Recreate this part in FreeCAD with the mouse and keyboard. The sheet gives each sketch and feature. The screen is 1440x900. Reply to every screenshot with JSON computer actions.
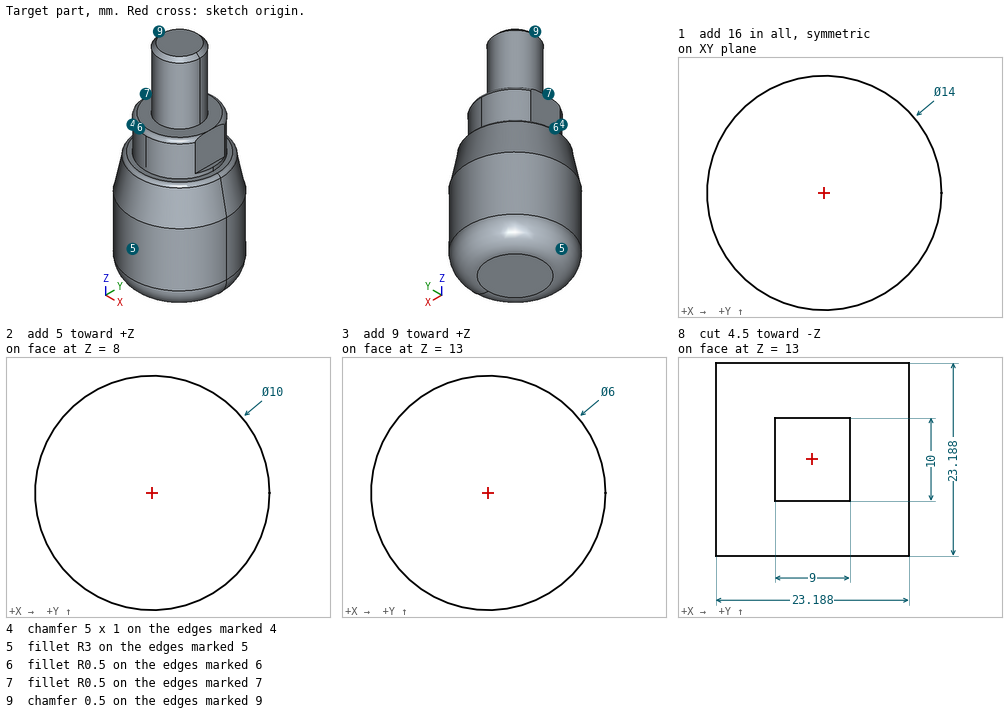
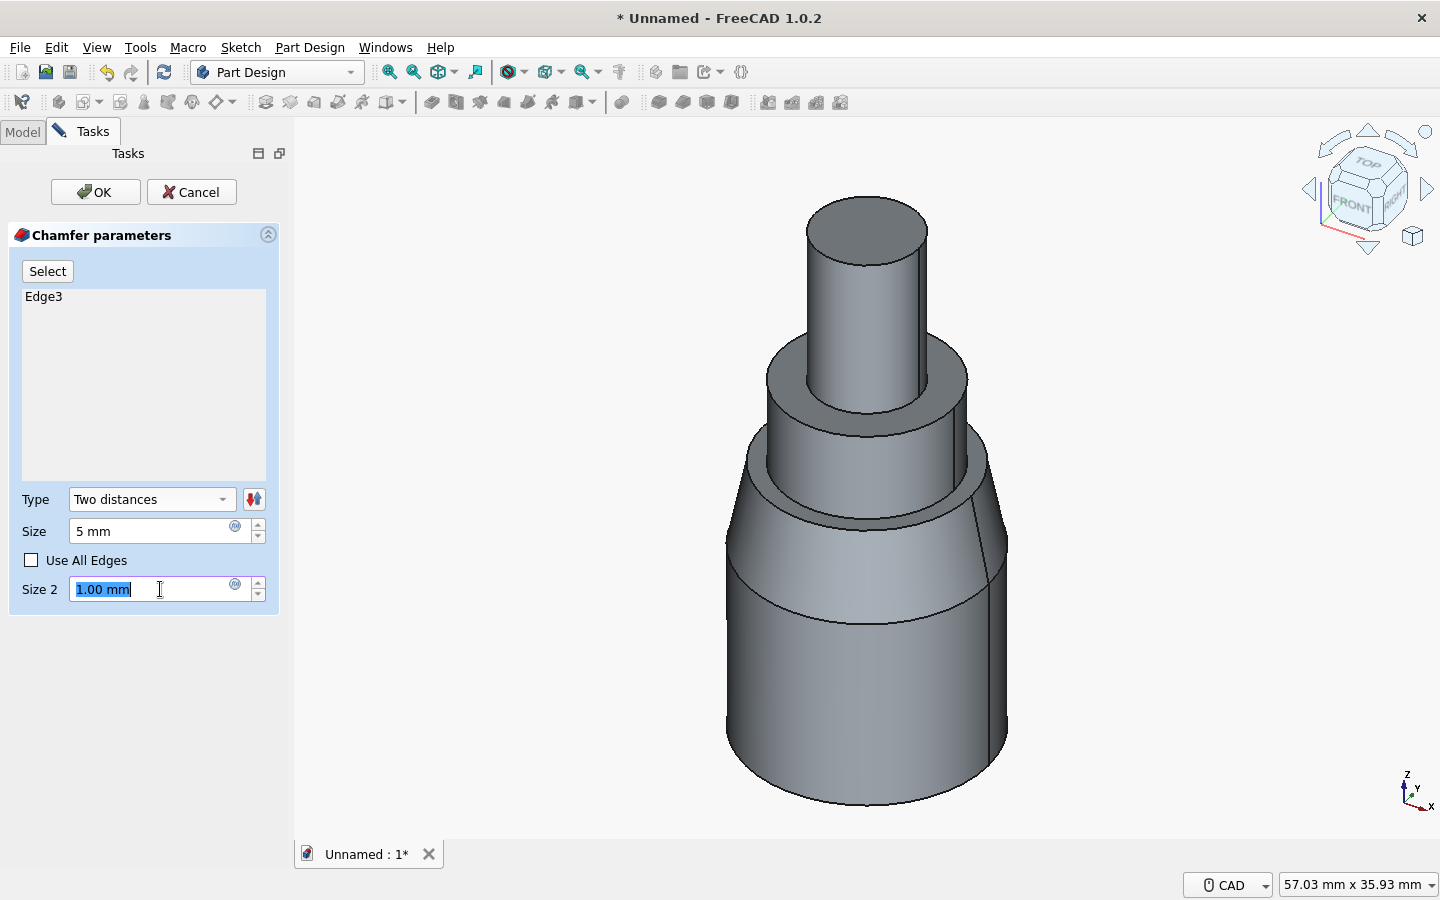
{"action": "type", "text": "1"}
{"action": "key", "text": "Tab"}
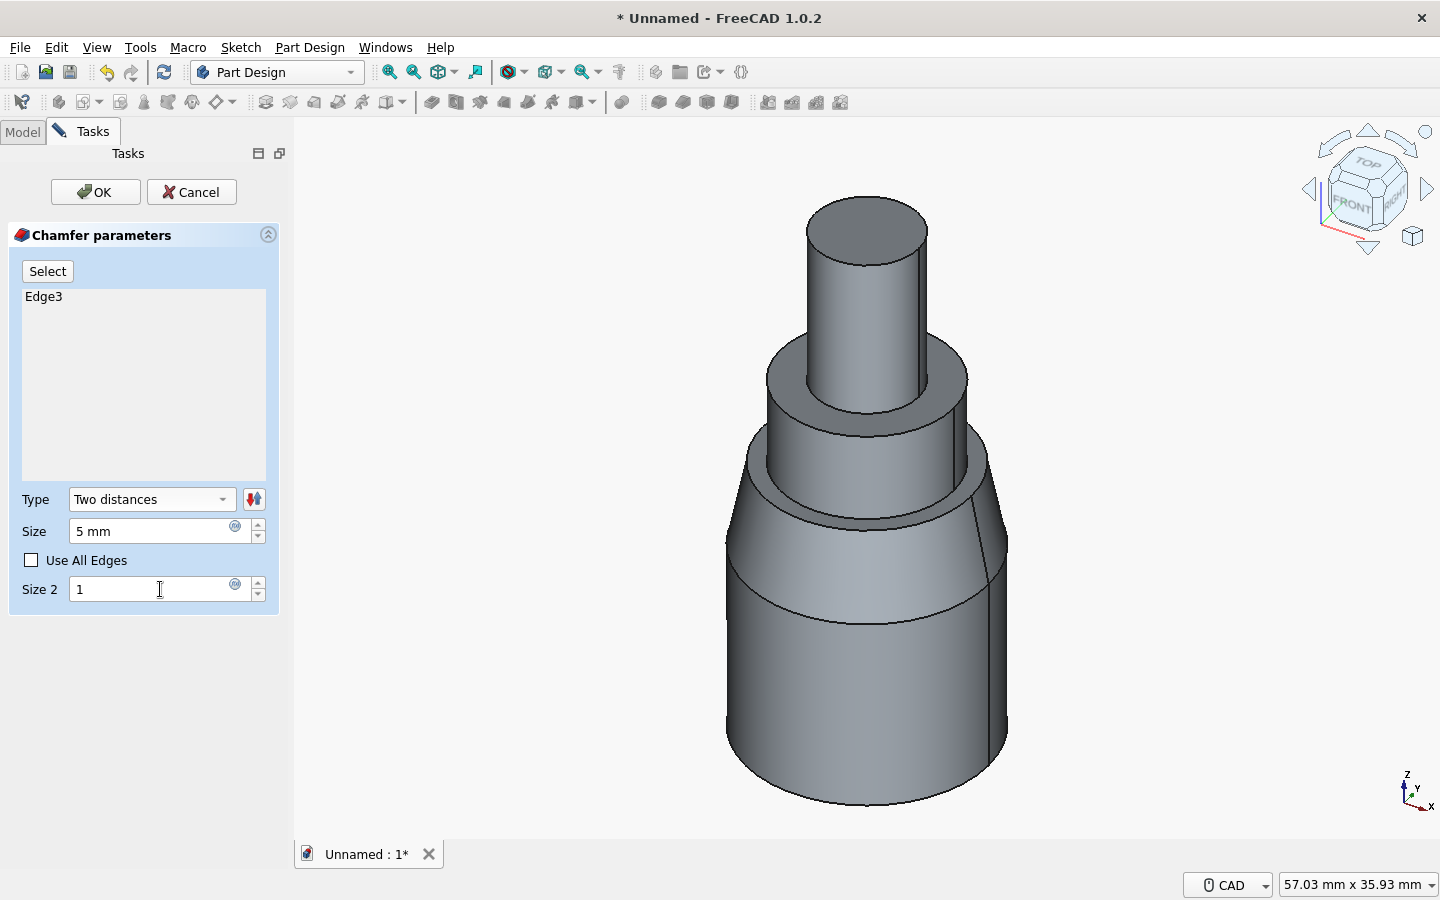
{"action": "left_click", "coordinate": [96, 192]}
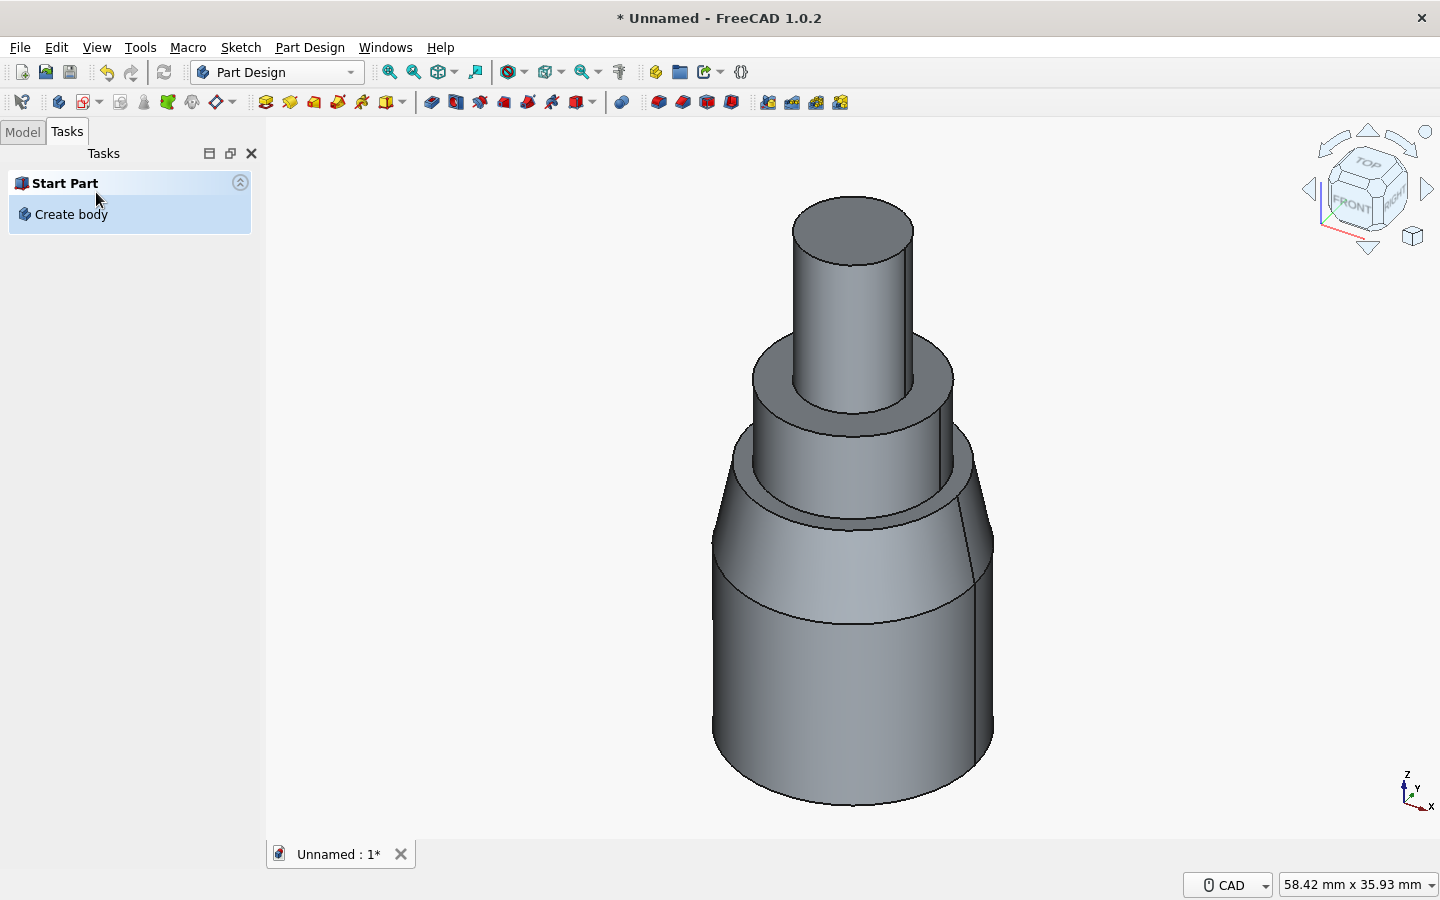
{"action": "key", "text": "0"}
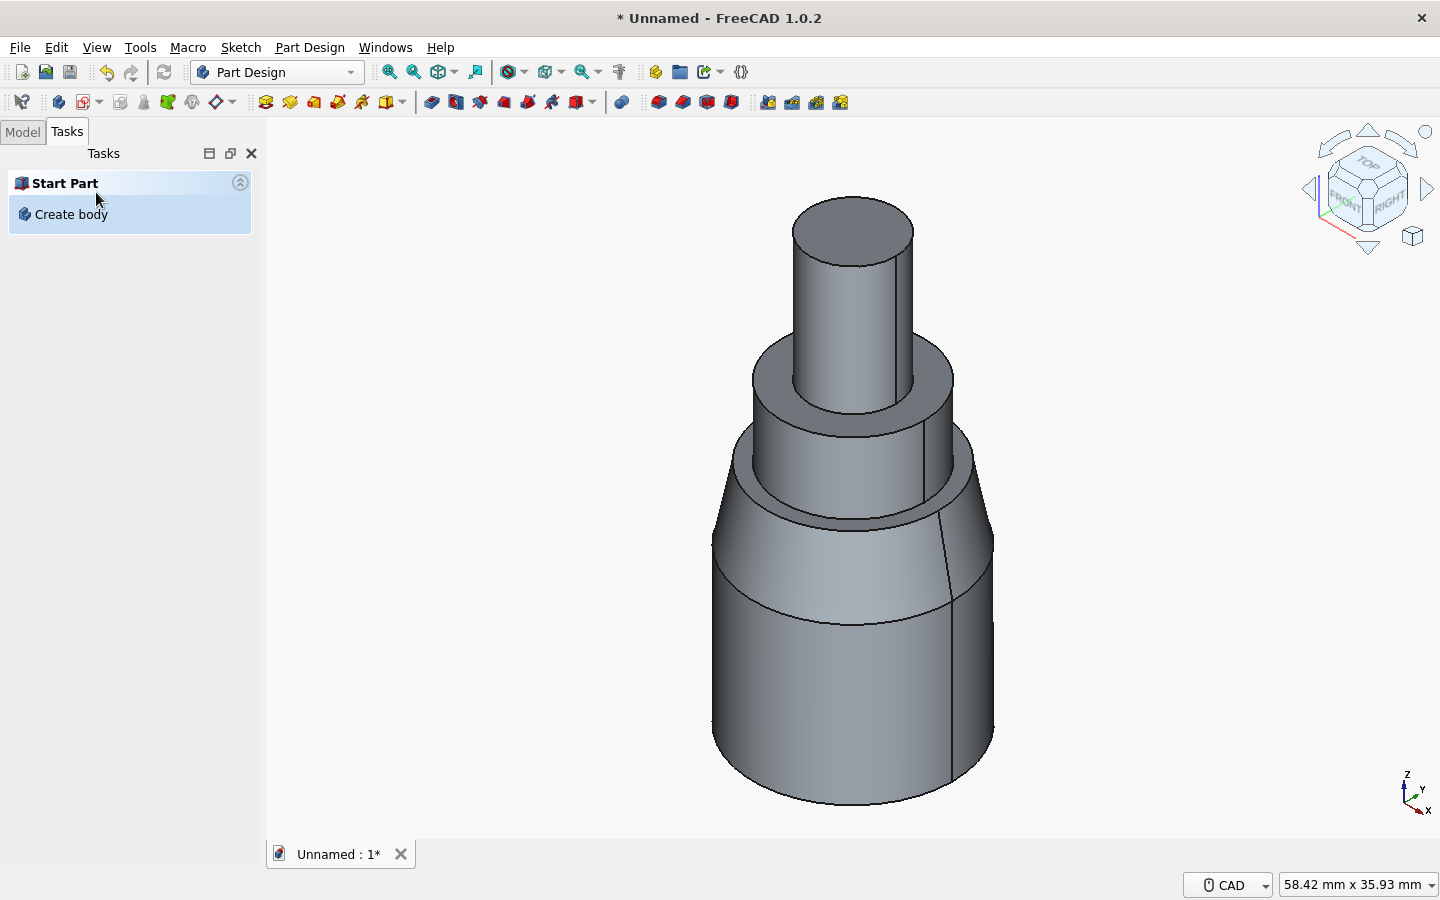
{"action": "key", "text": "v f"}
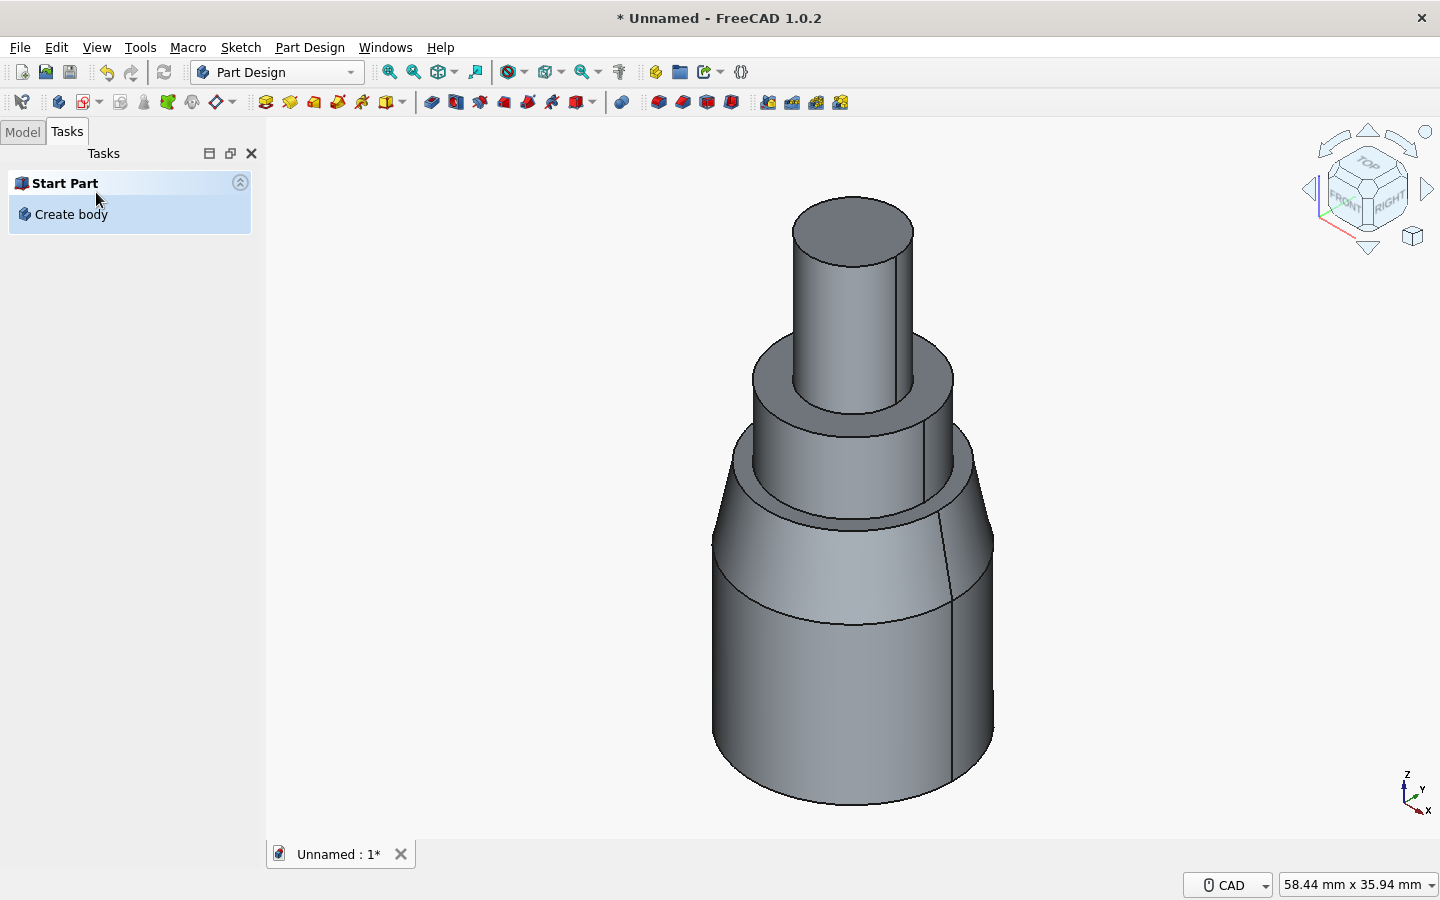
{"action": "left_click", "coordinate": [969, 769]}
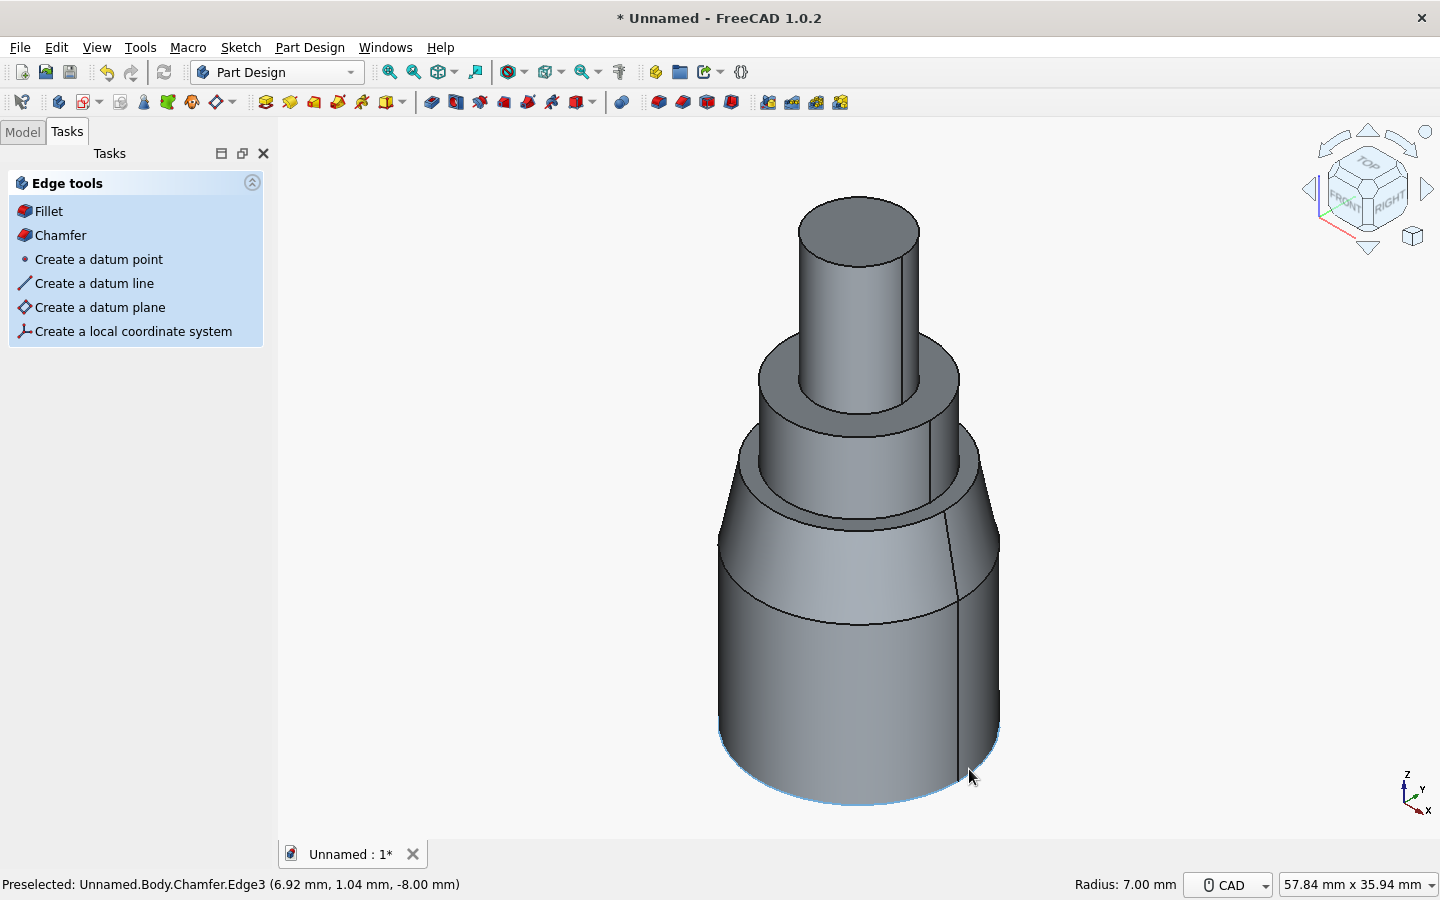
{"action": "left_click", "coordinate": [660, 102]}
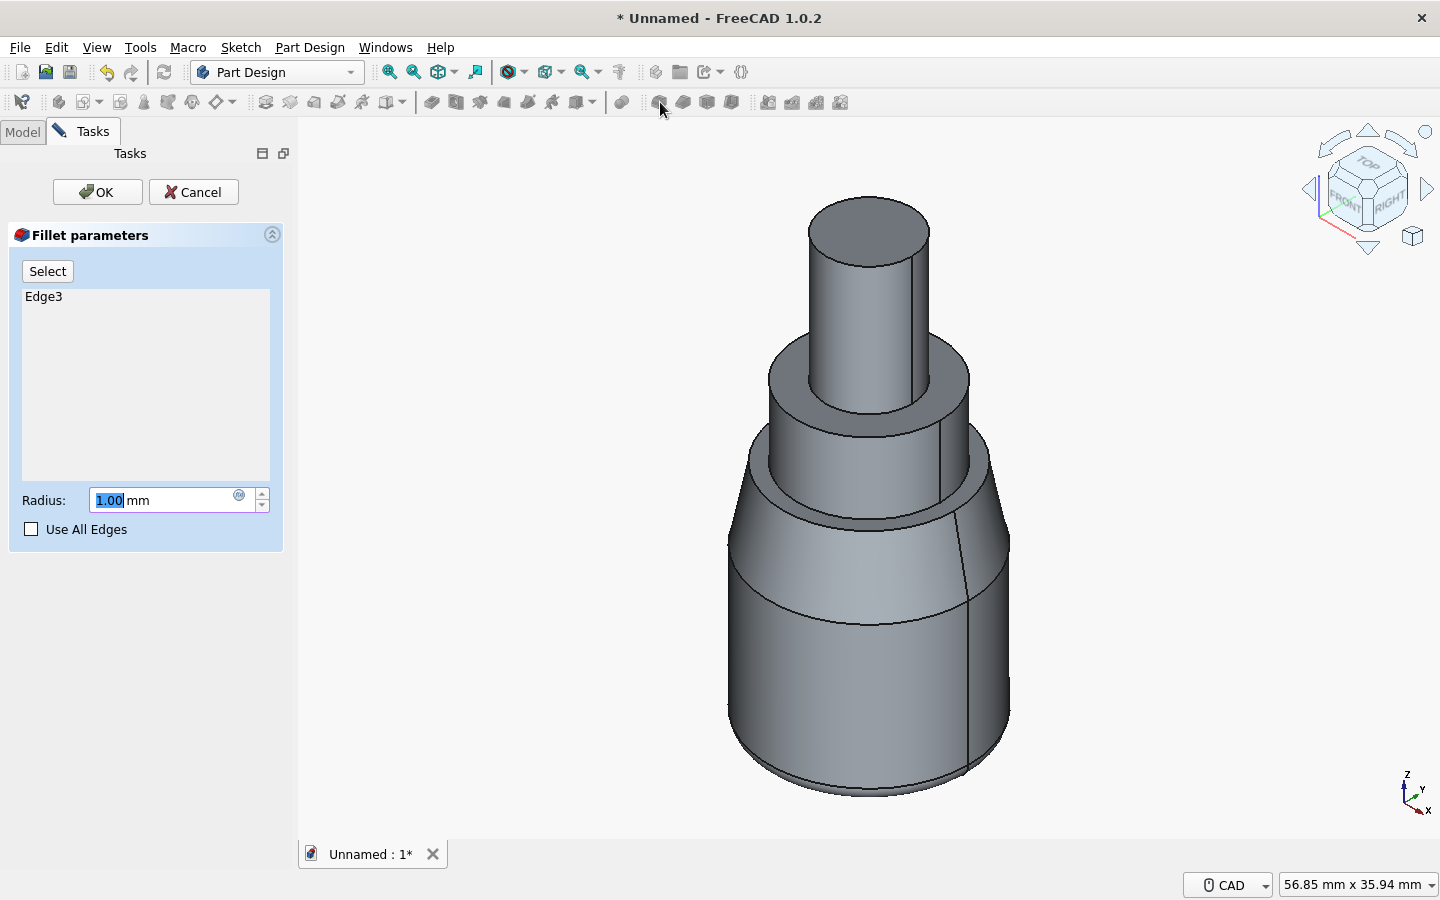
{"action": "type", "text": "3"}
{"action": "key", "text": "Tab"}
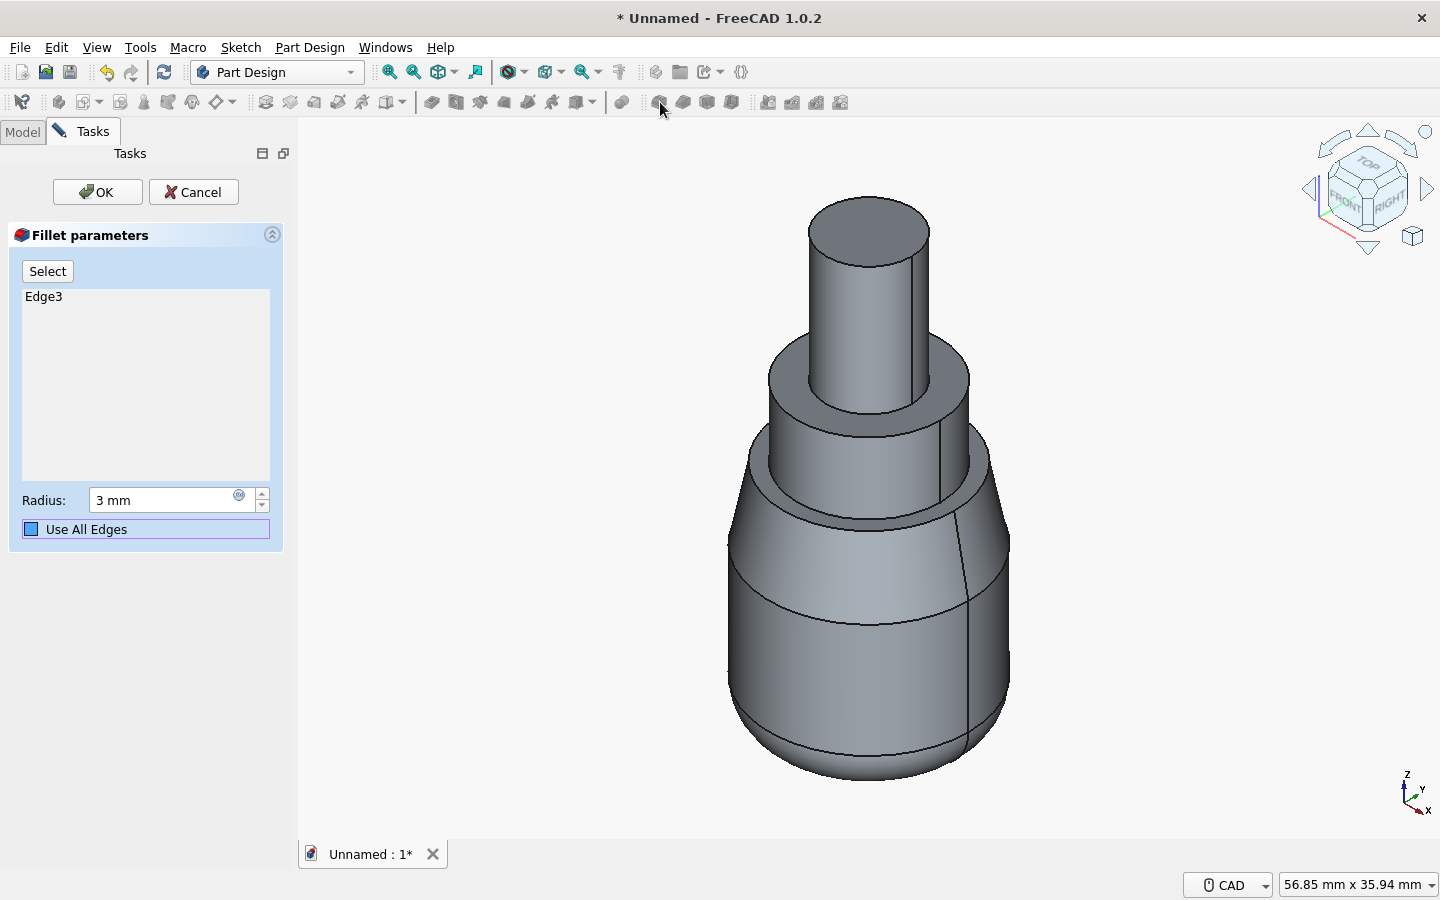
{"action": "left_click", "coordinate": [98, 192]}